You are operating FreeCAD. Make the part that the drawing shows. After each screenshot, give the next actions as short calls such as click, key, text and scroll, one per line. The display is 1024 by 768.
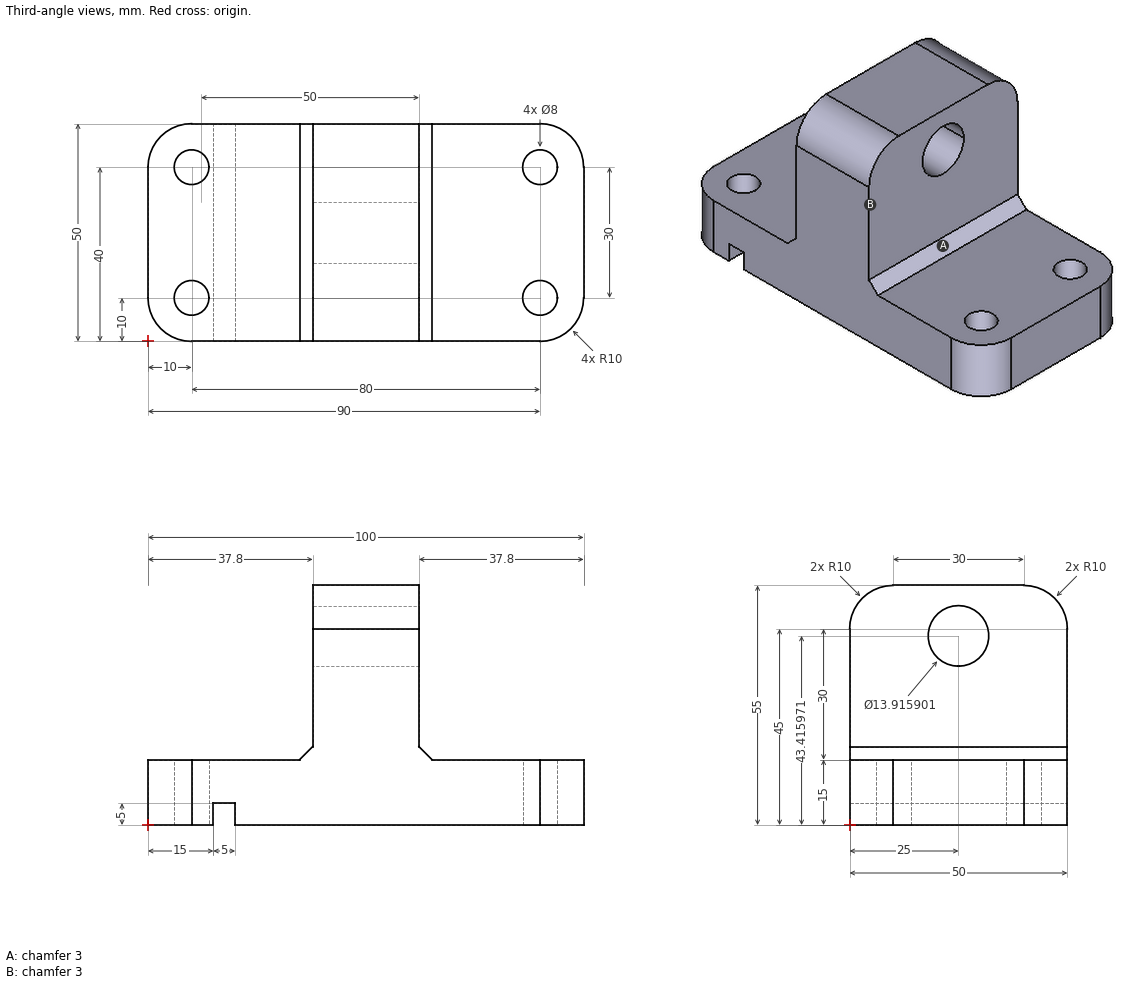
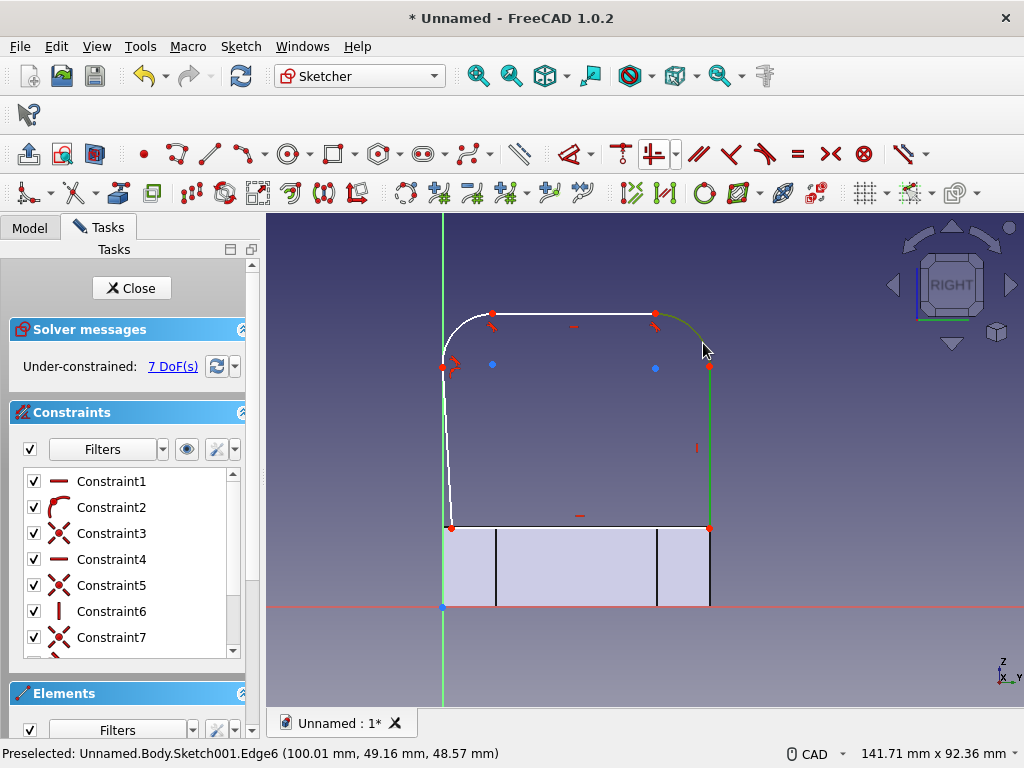
click(765, 154)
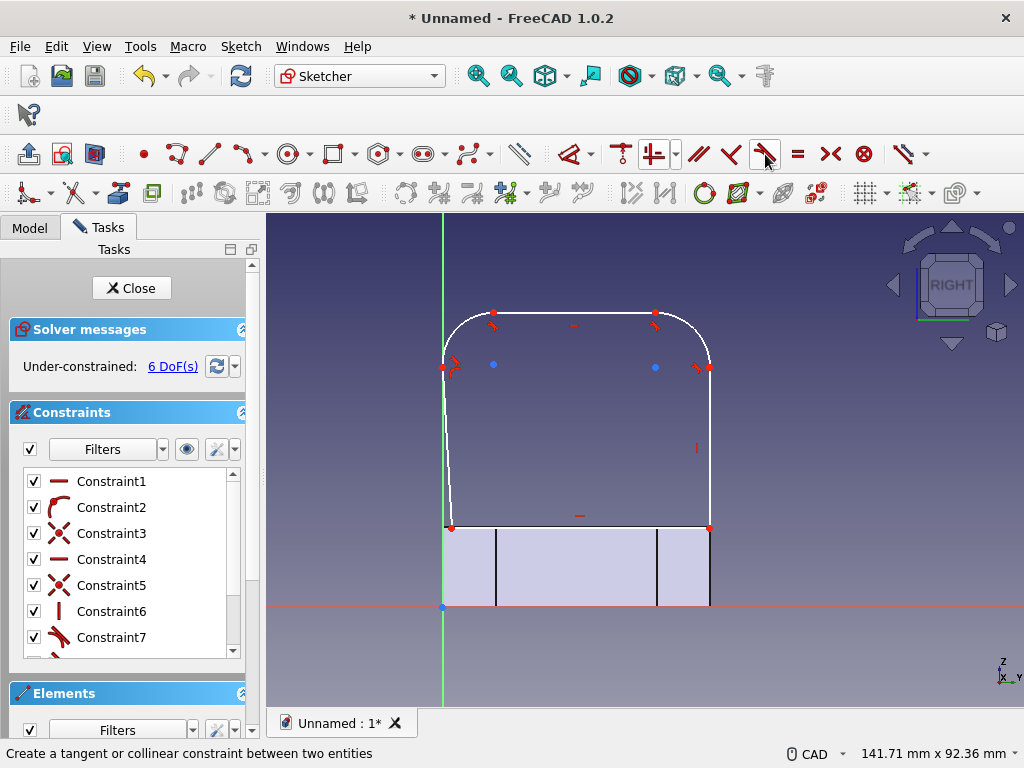
click(446, 415)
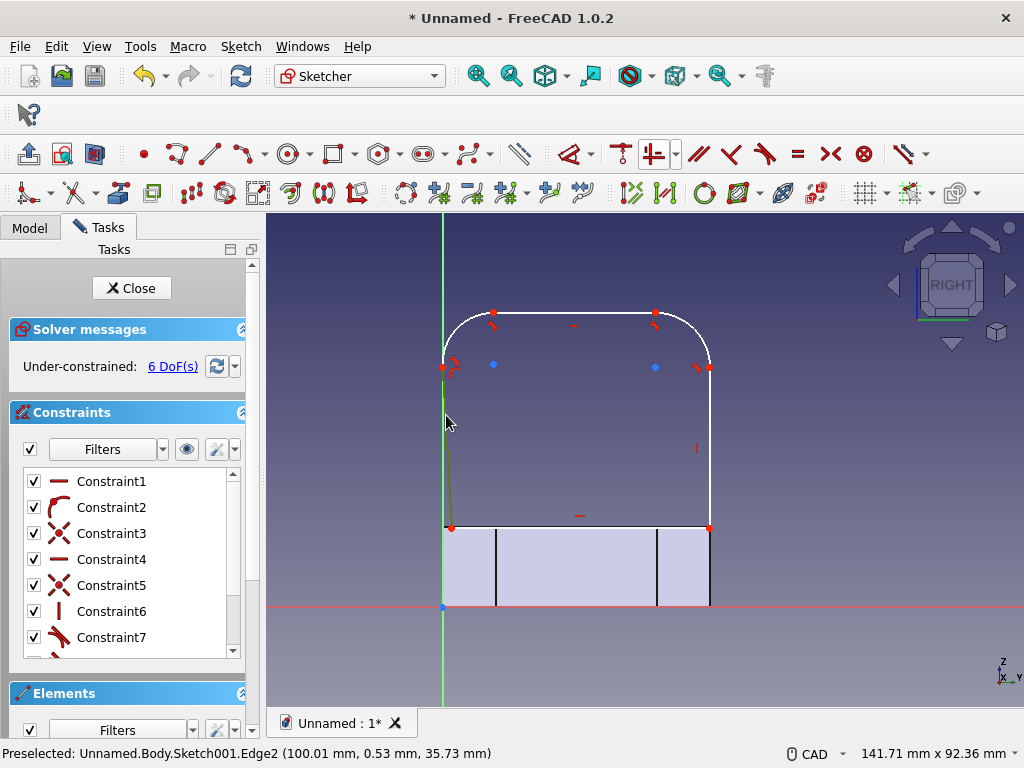
click(676, 154)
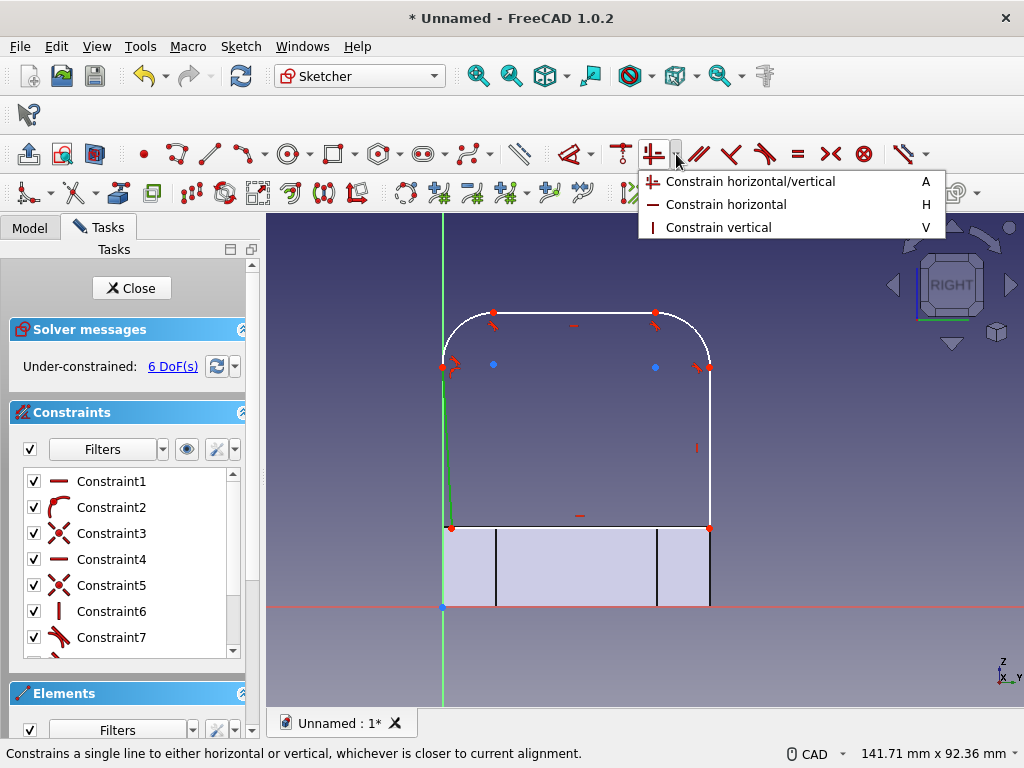
click(792, 228)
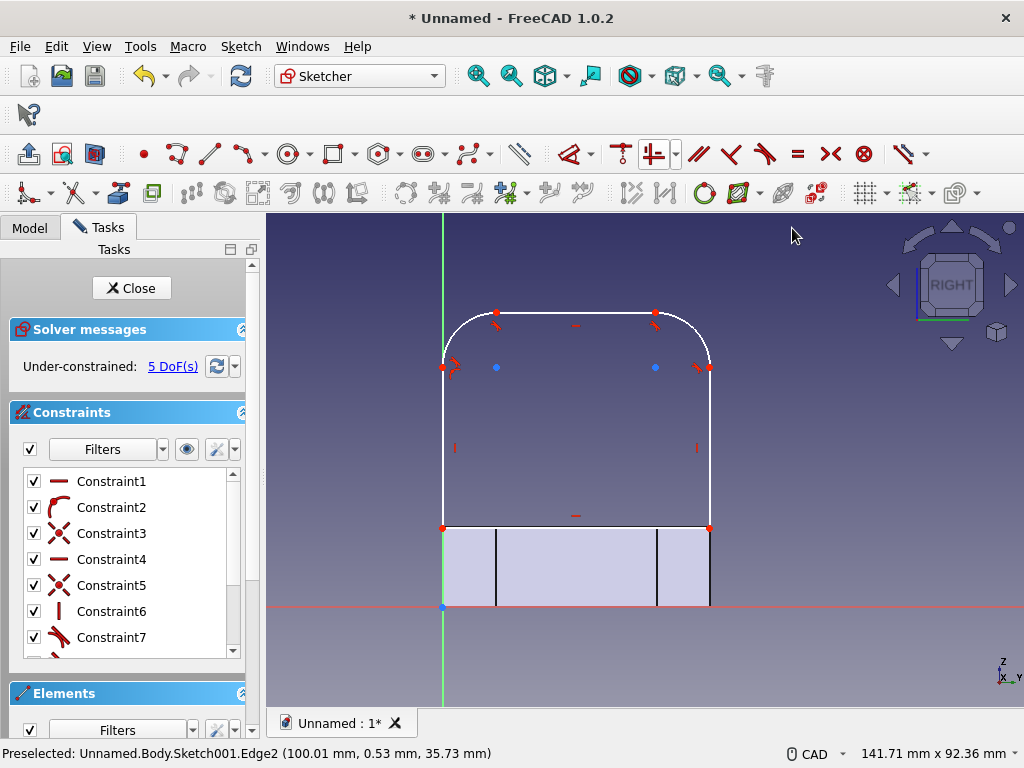
click(472, 319)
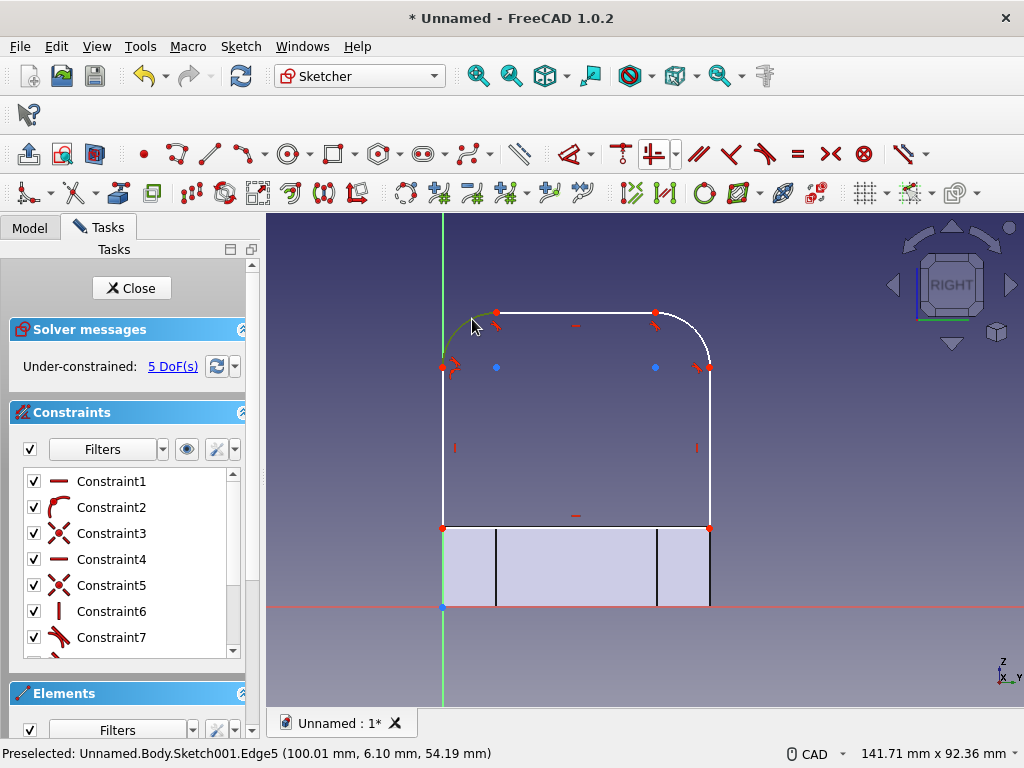
click(704, 343)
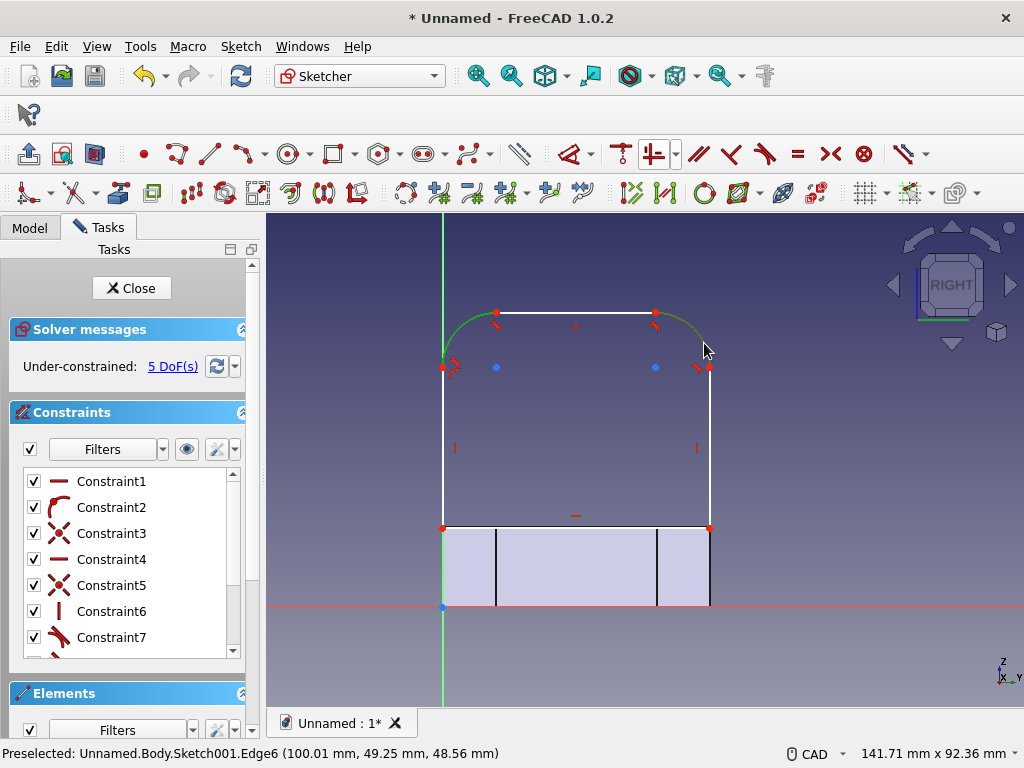
click(798, 154)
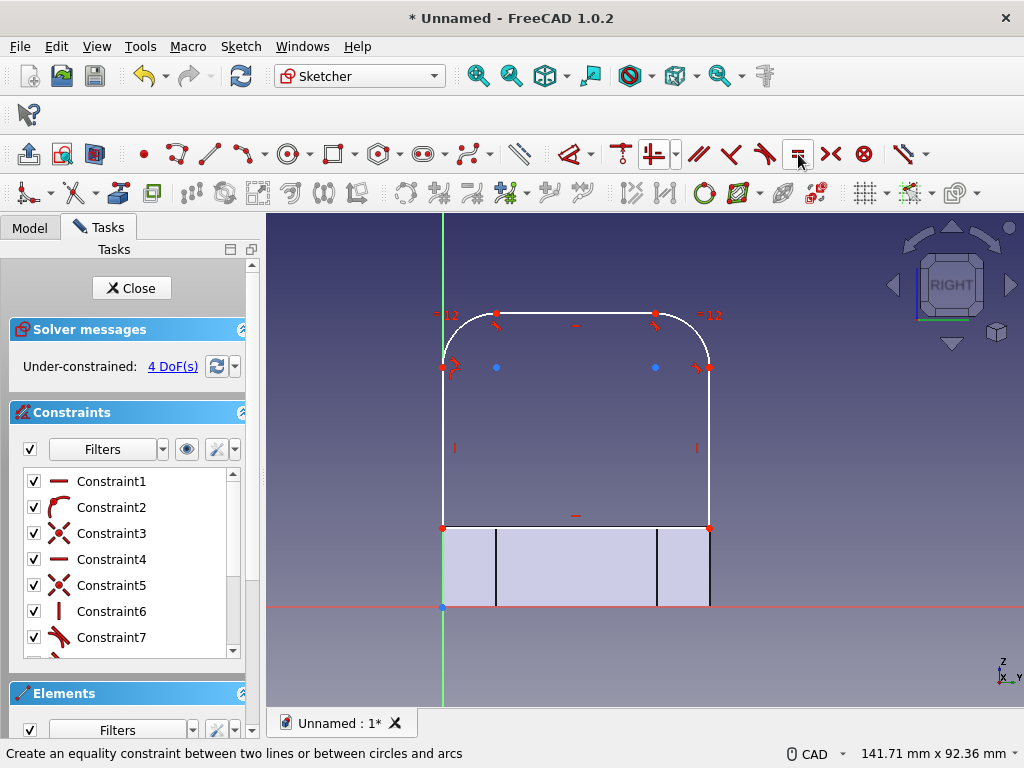
click(568, 154)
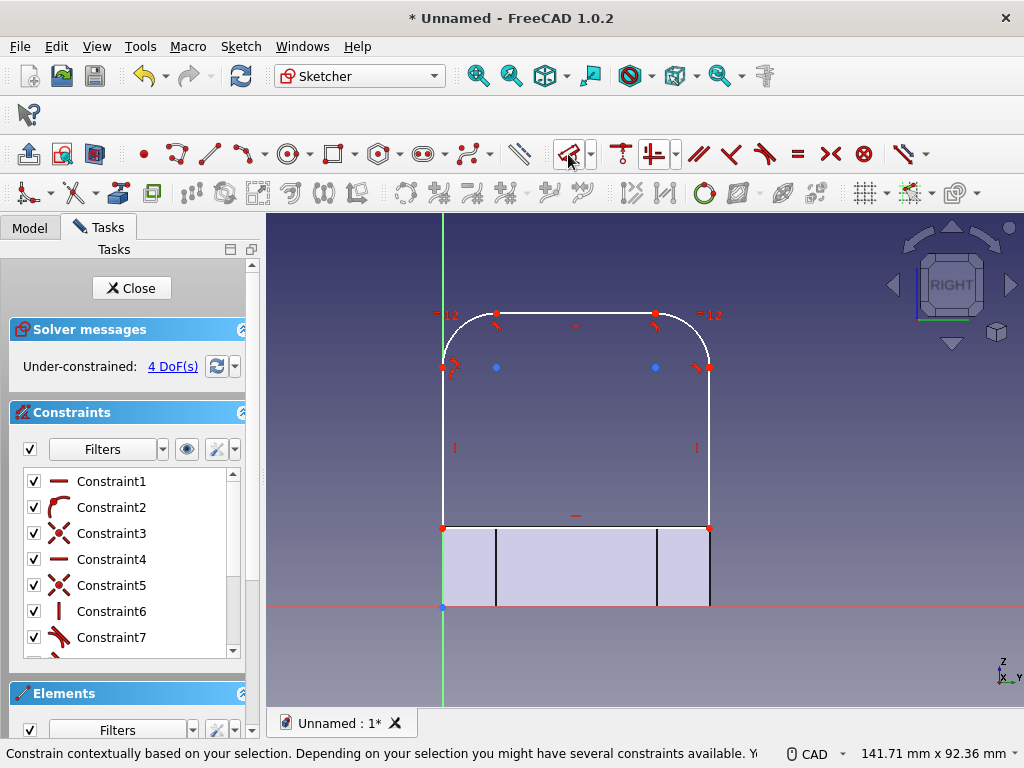
click(472, 319)
click(457, 291)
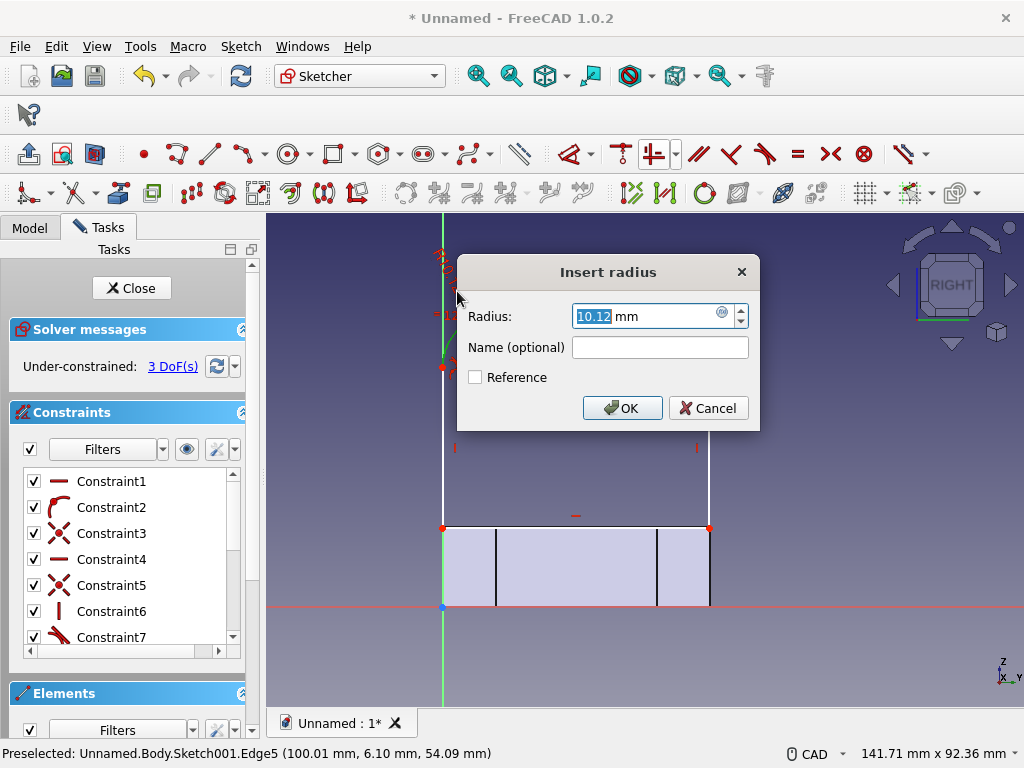
text(10)
key(Return)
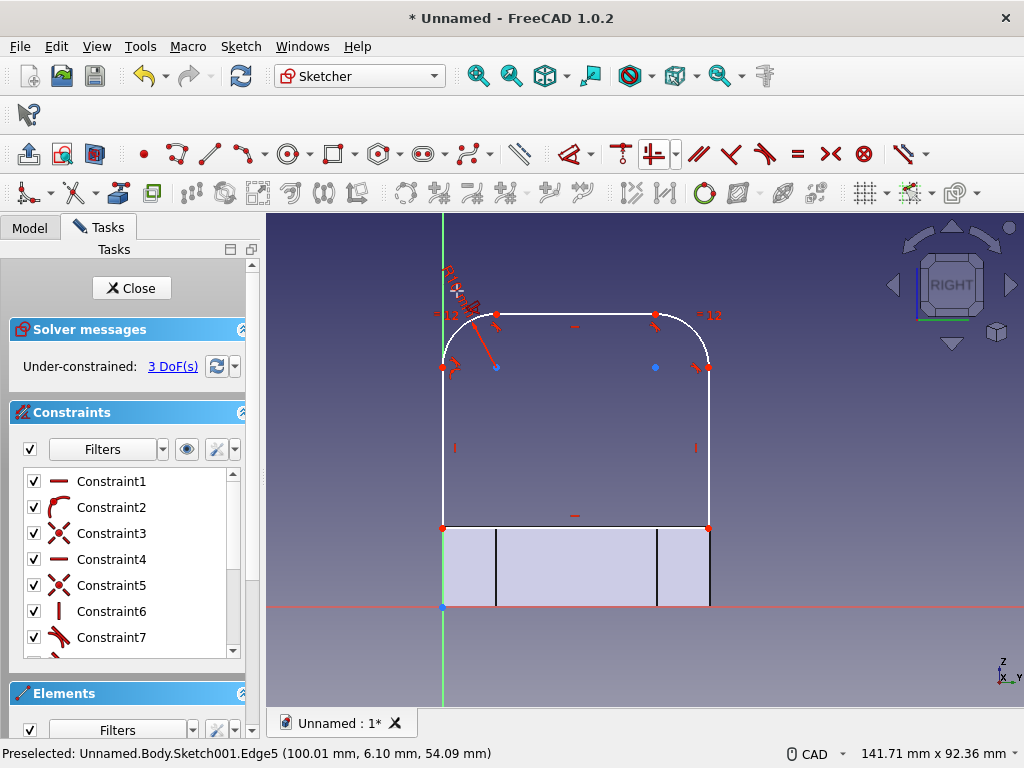
click(608, 314)
click(576, 280)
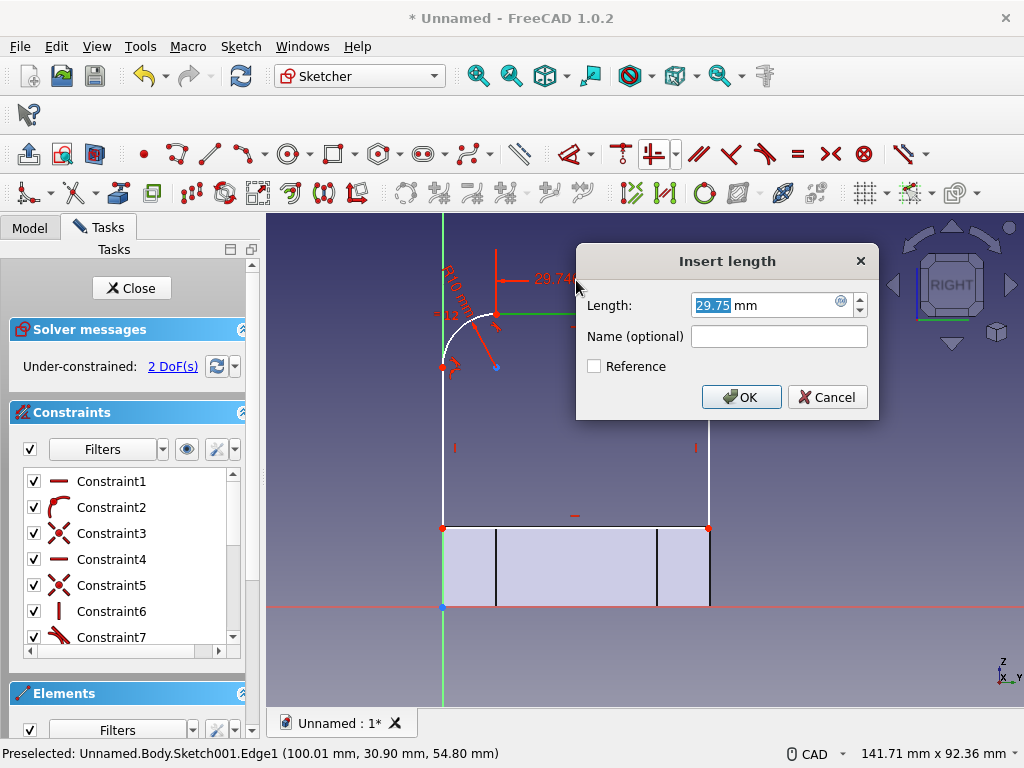
text(30)
key(Return)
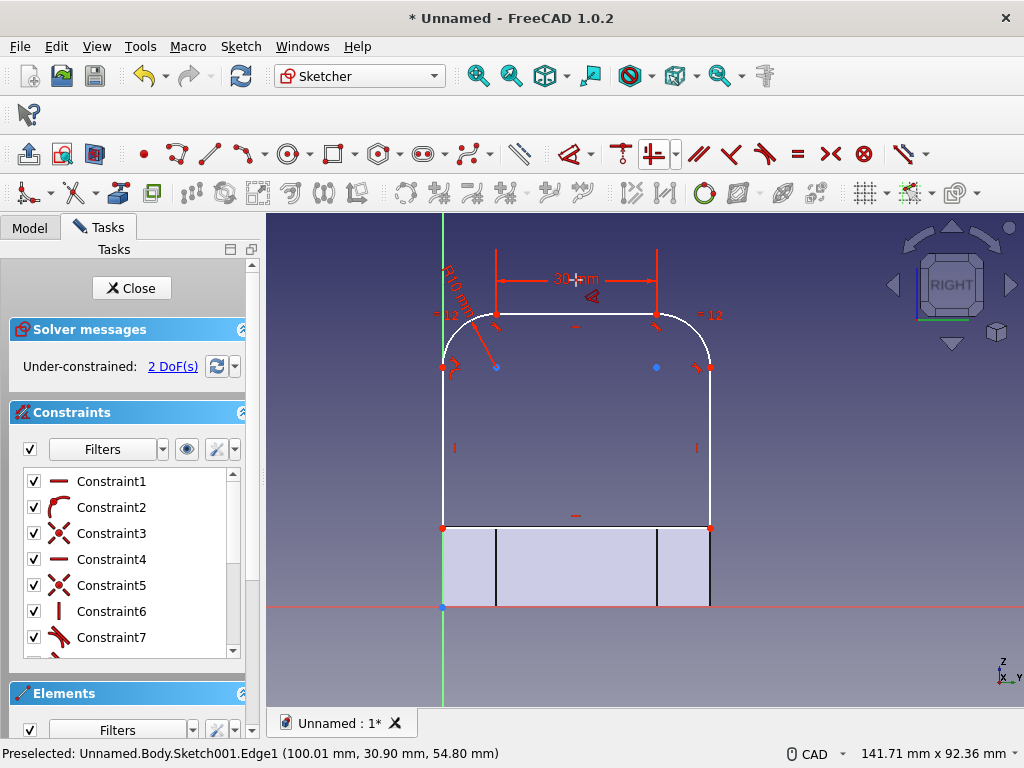
click(443, 416)
click(409, 448)